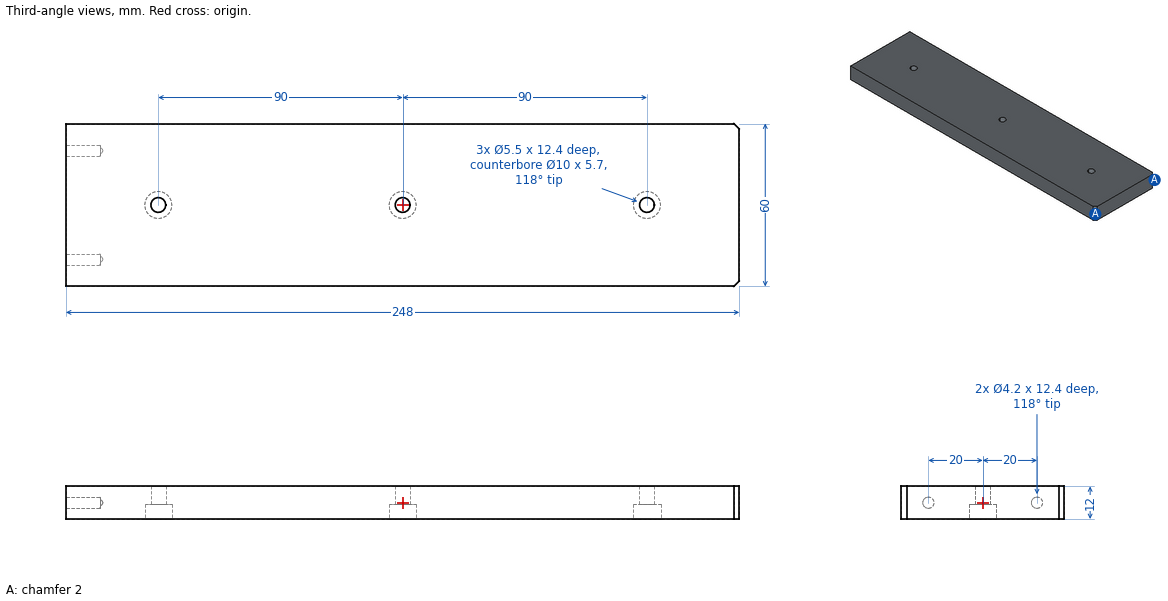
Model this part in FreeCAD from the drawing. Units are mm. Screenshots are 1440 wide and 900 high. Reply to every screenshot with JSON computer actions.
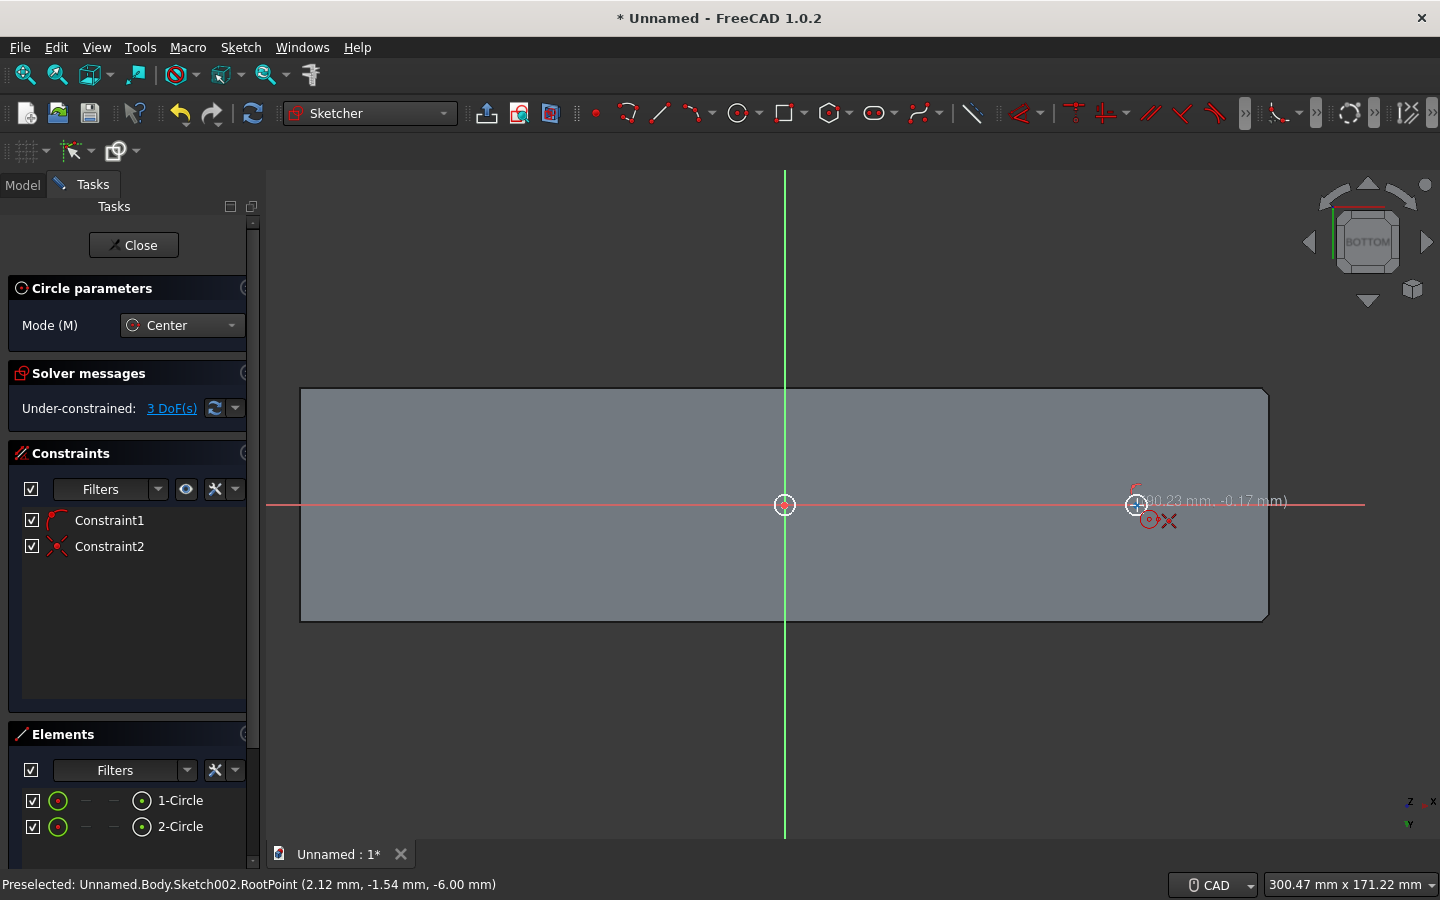
{"action": "scroll", "coordinate": [433, 505], "scroll_direction": "up", "scroll_amount": 4}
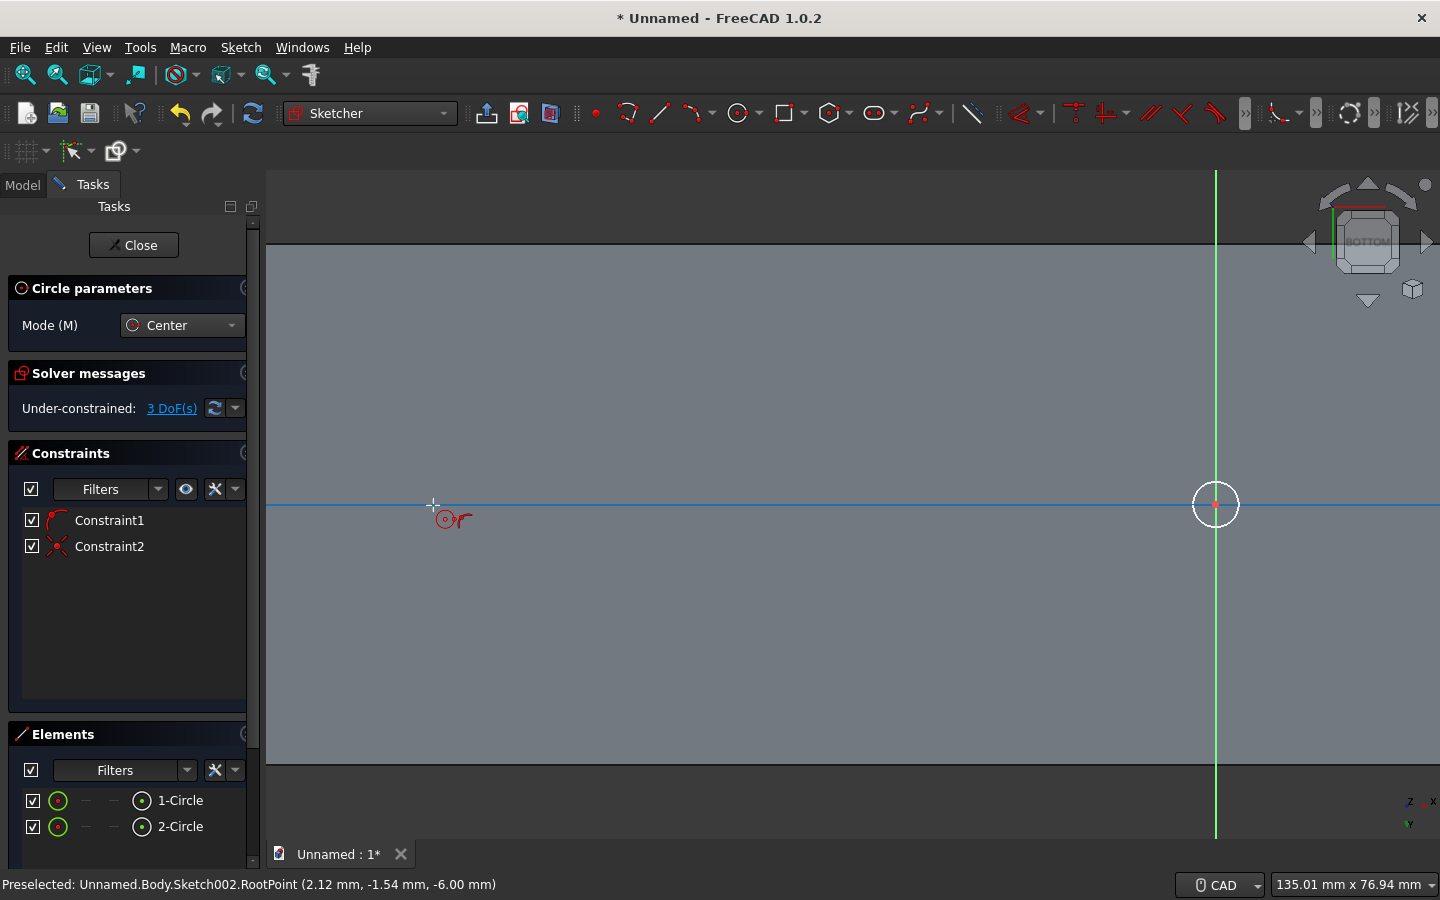
{"action": "left_click", "coordinate": [433, 504]}
{"action": "left_click", "coordinate": [450, 488]}
{"action": "key", "text": "Escape"}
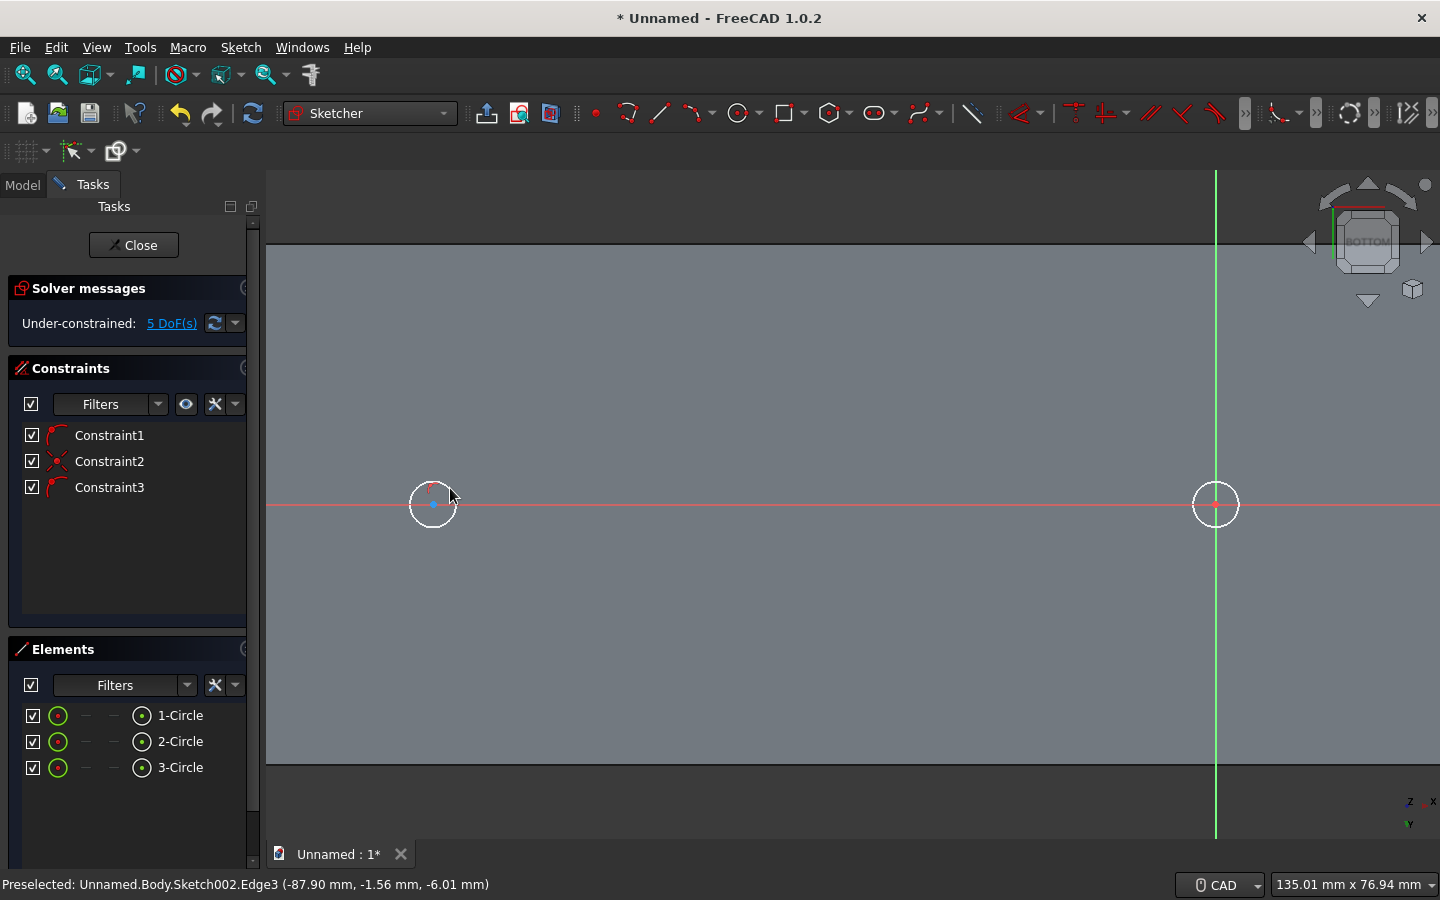
{"action": "scroll", "coordinate": [432, 505], "scroll_direction": "down", "scroll_amount": 4}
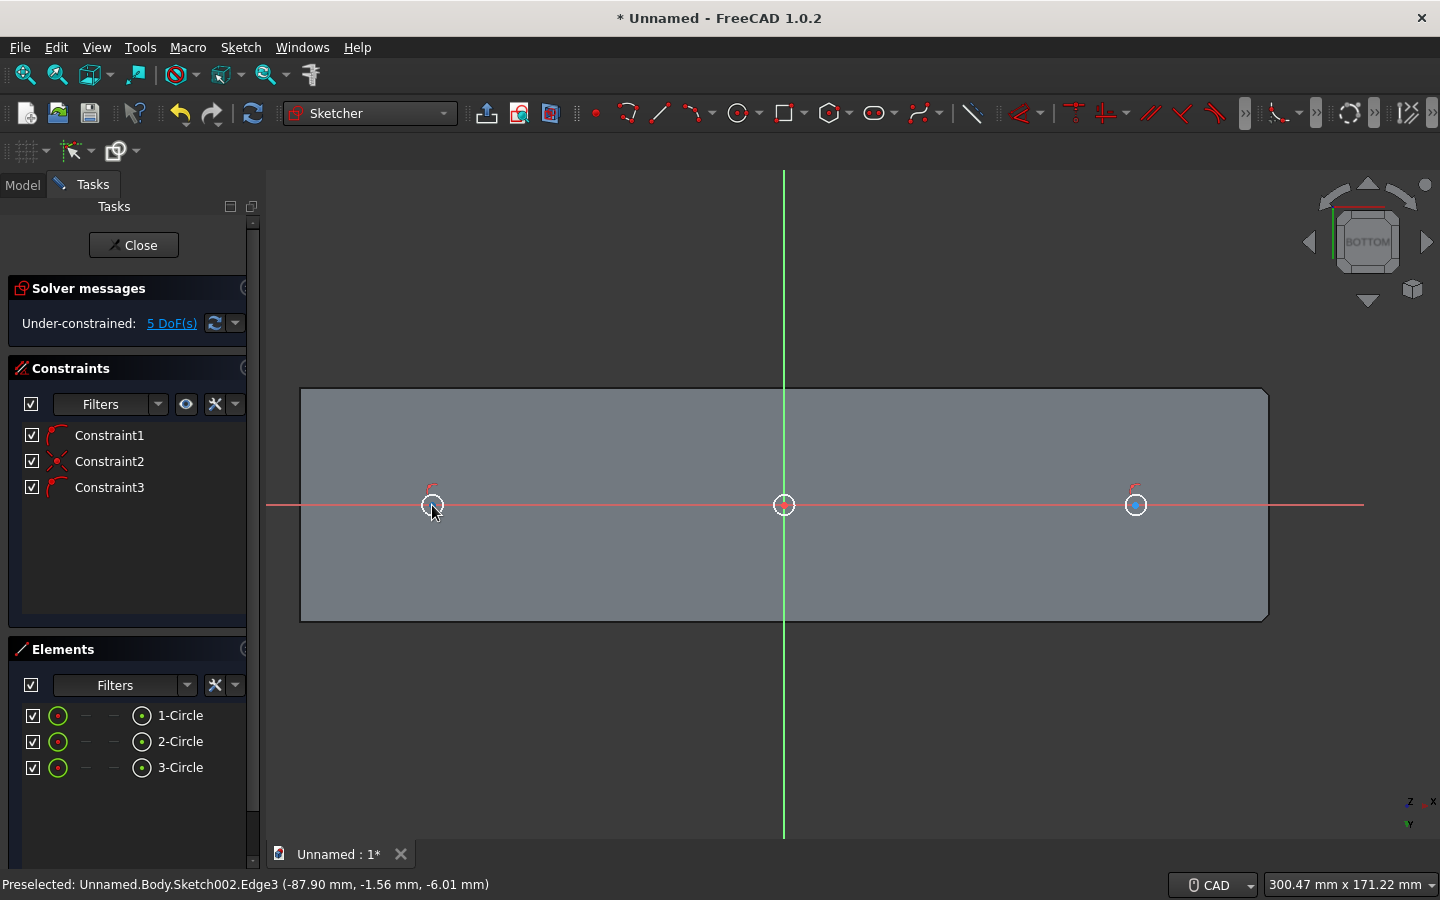
{"action": "scroll", "coordinate": [1143, 498], "scroll_direction": "up", "scroll_amount": 4}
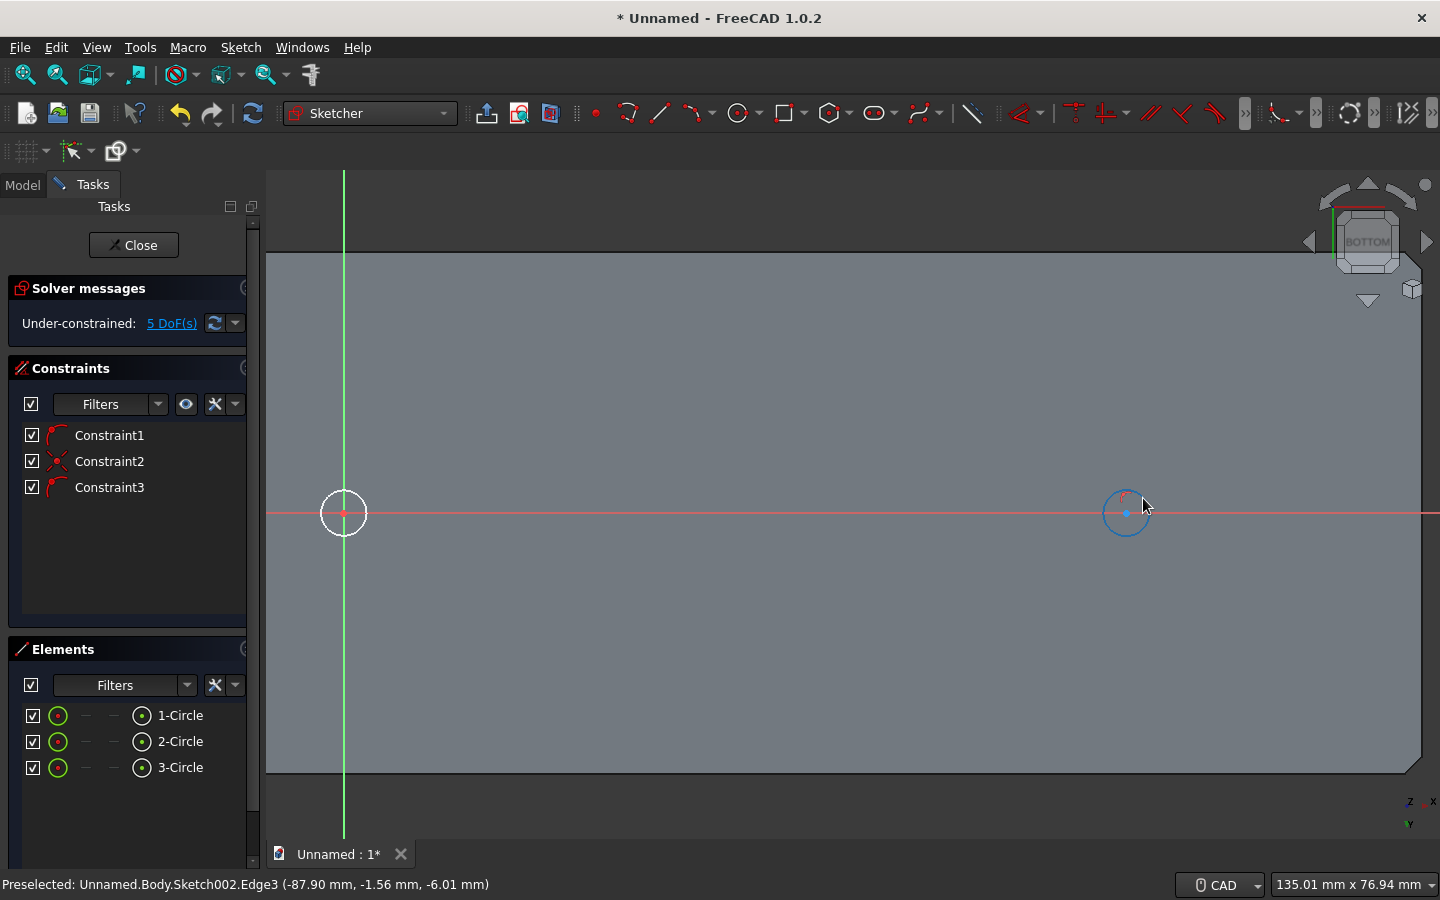
{"action": "left_click", "coordinate": [1143, 497]}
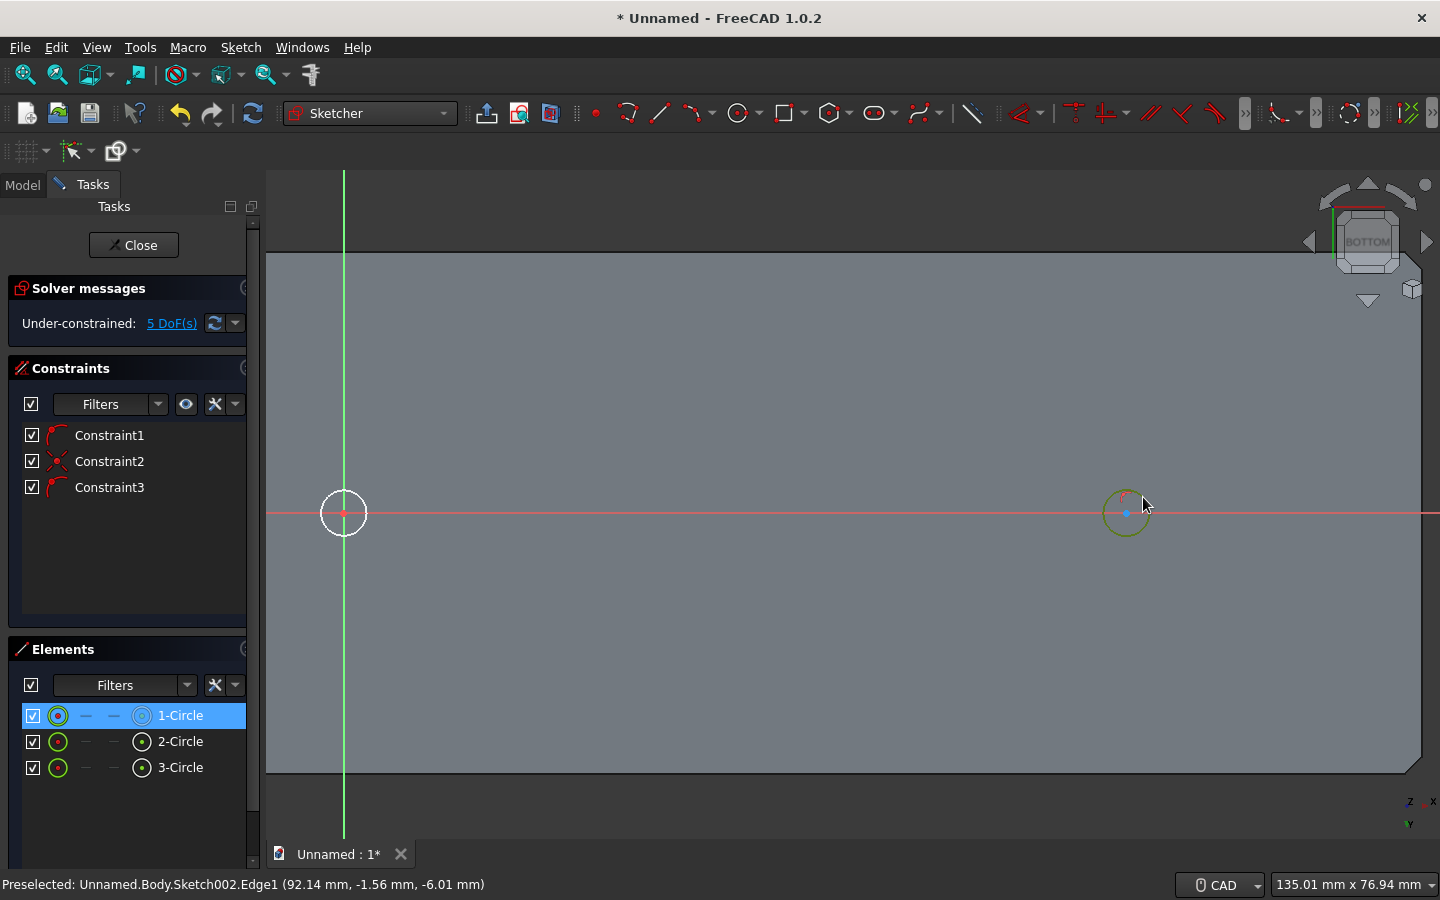
{"action": "left_click", "coordinate": [360, 497]}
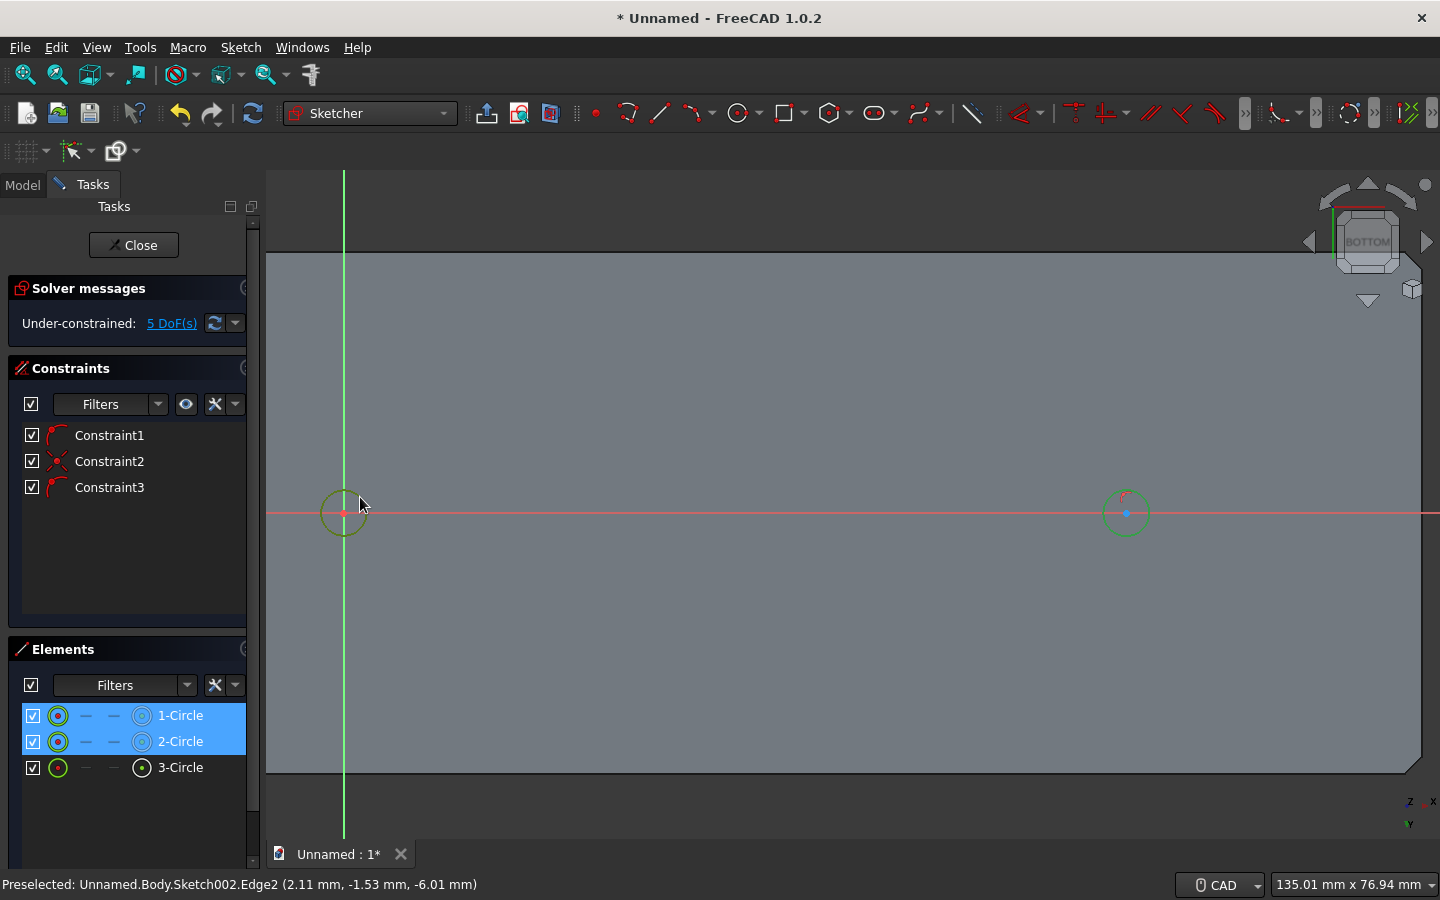
{"action": "scroll", "coordinate": [1144, 497], "scroll_direction": "down", "scroll_amount": 4}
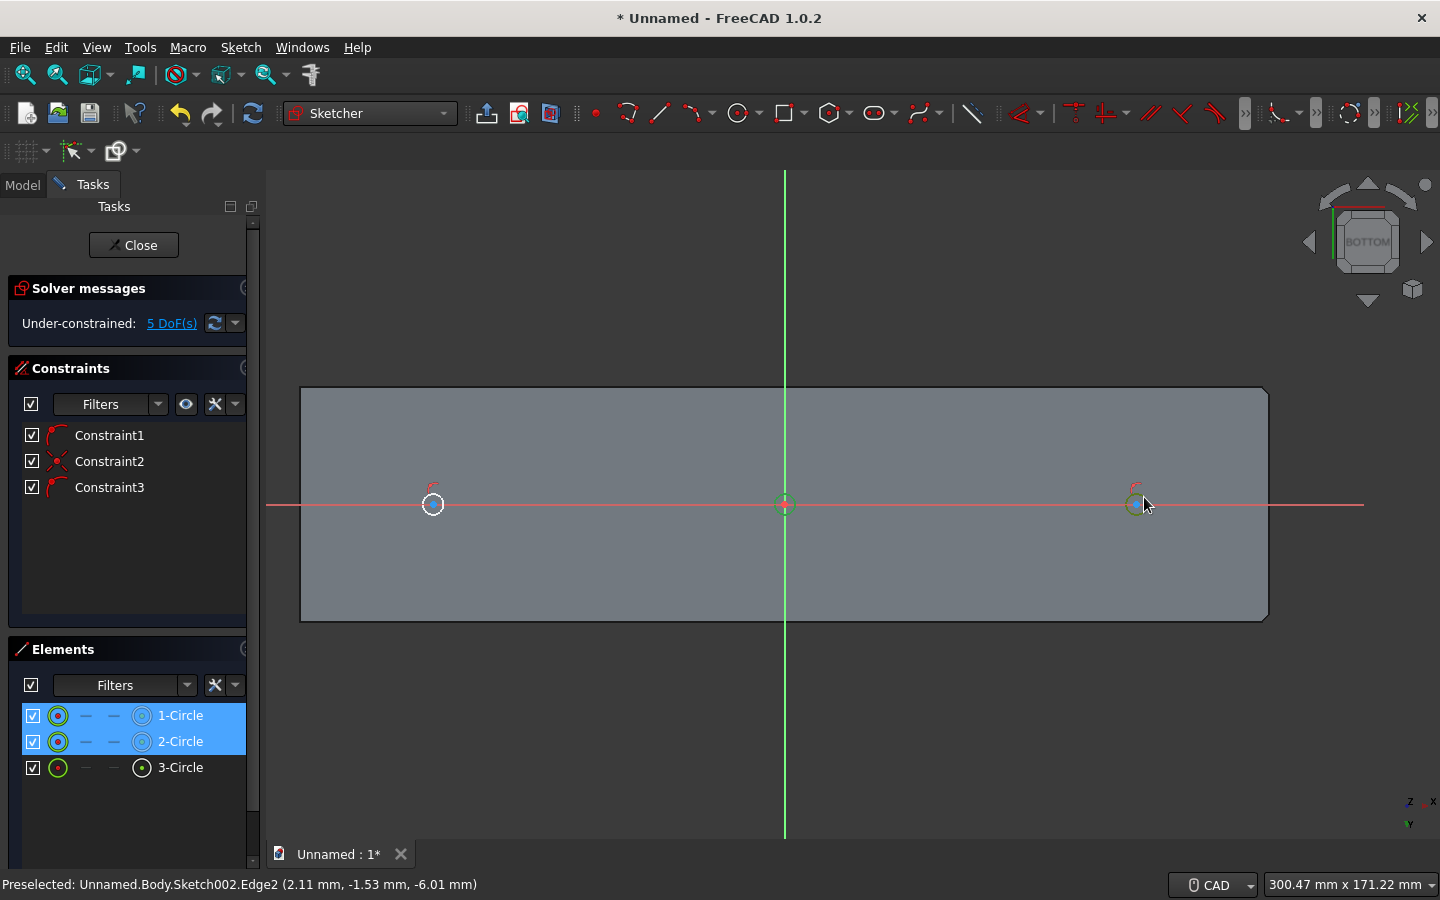
{"action": "scroll", "coordinate": [440, 497], "scroll_direction": "up", "scroll_amount": 4}